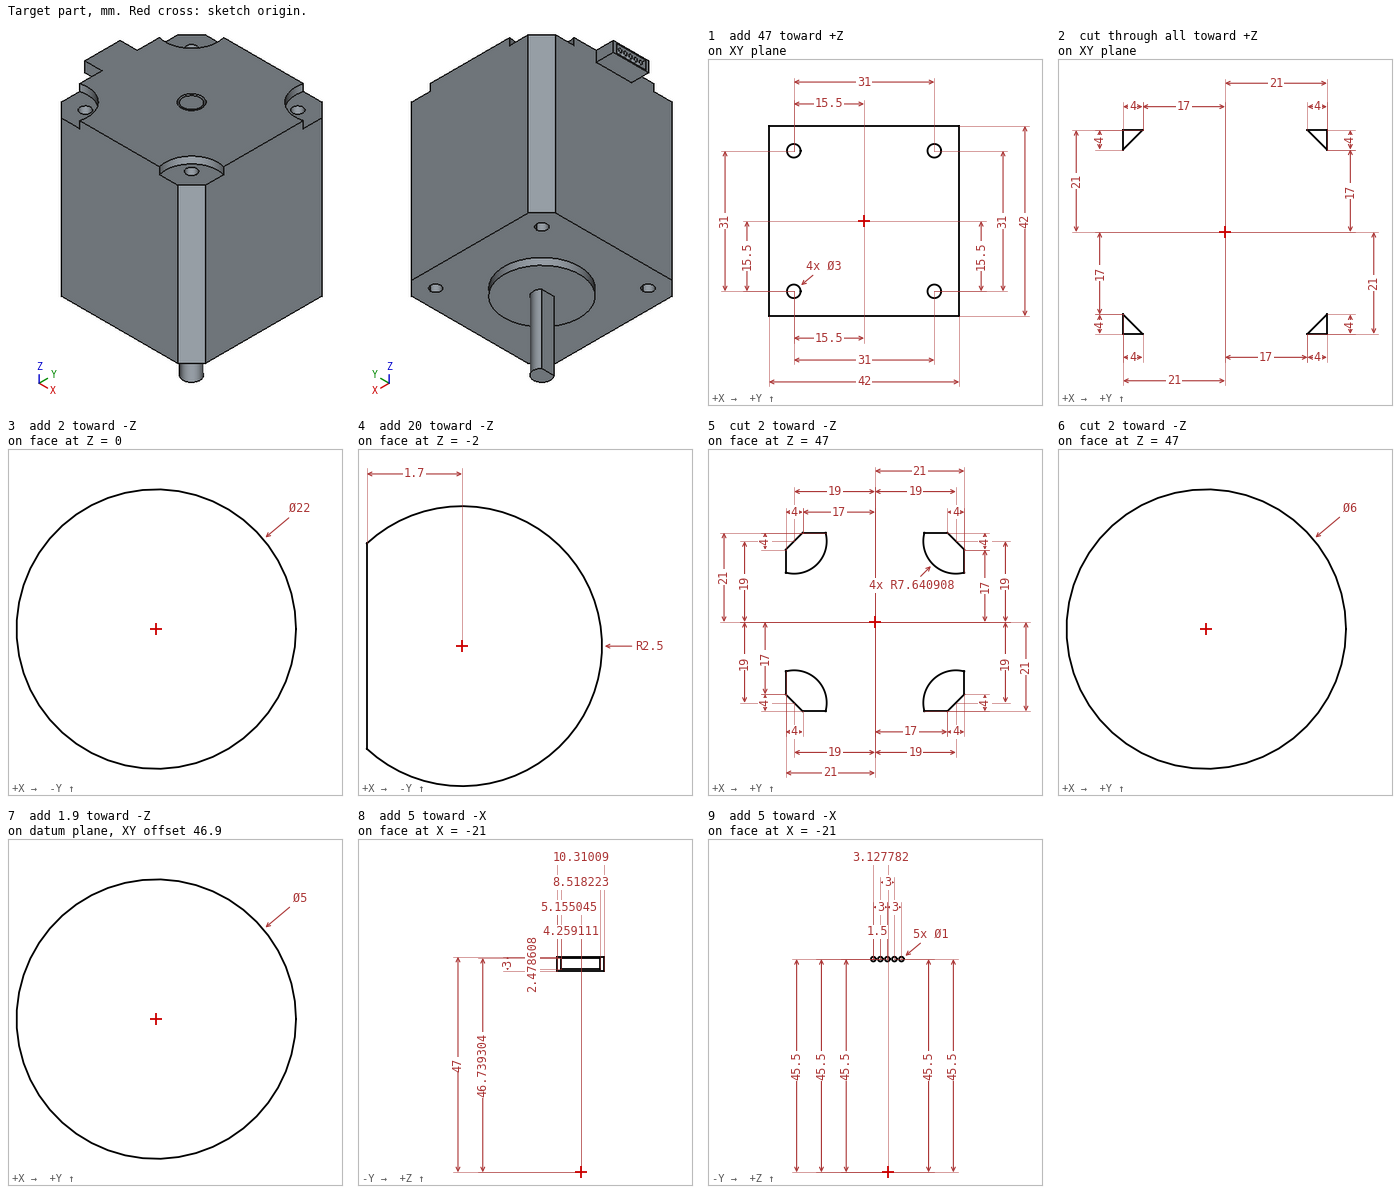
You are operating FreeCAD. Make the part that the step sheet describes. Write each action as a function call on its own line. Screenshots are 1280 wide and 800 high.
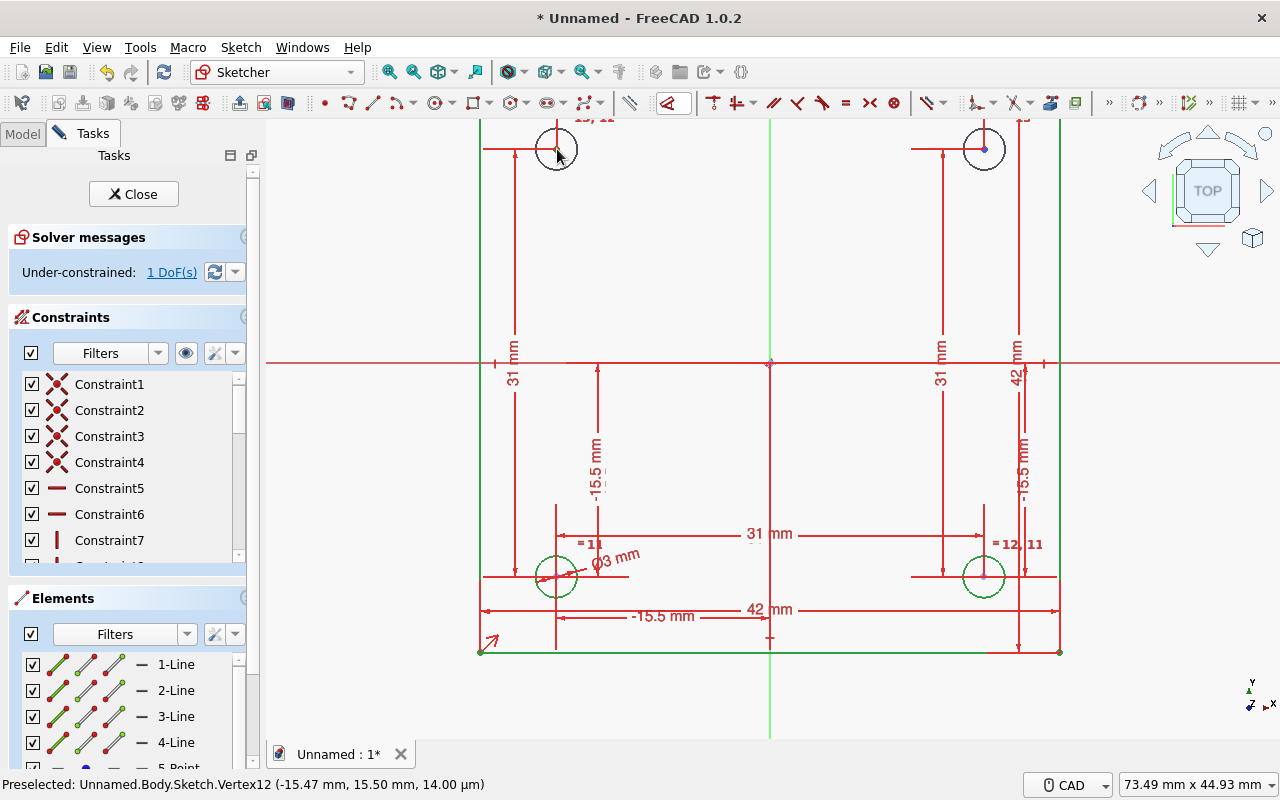
key(l)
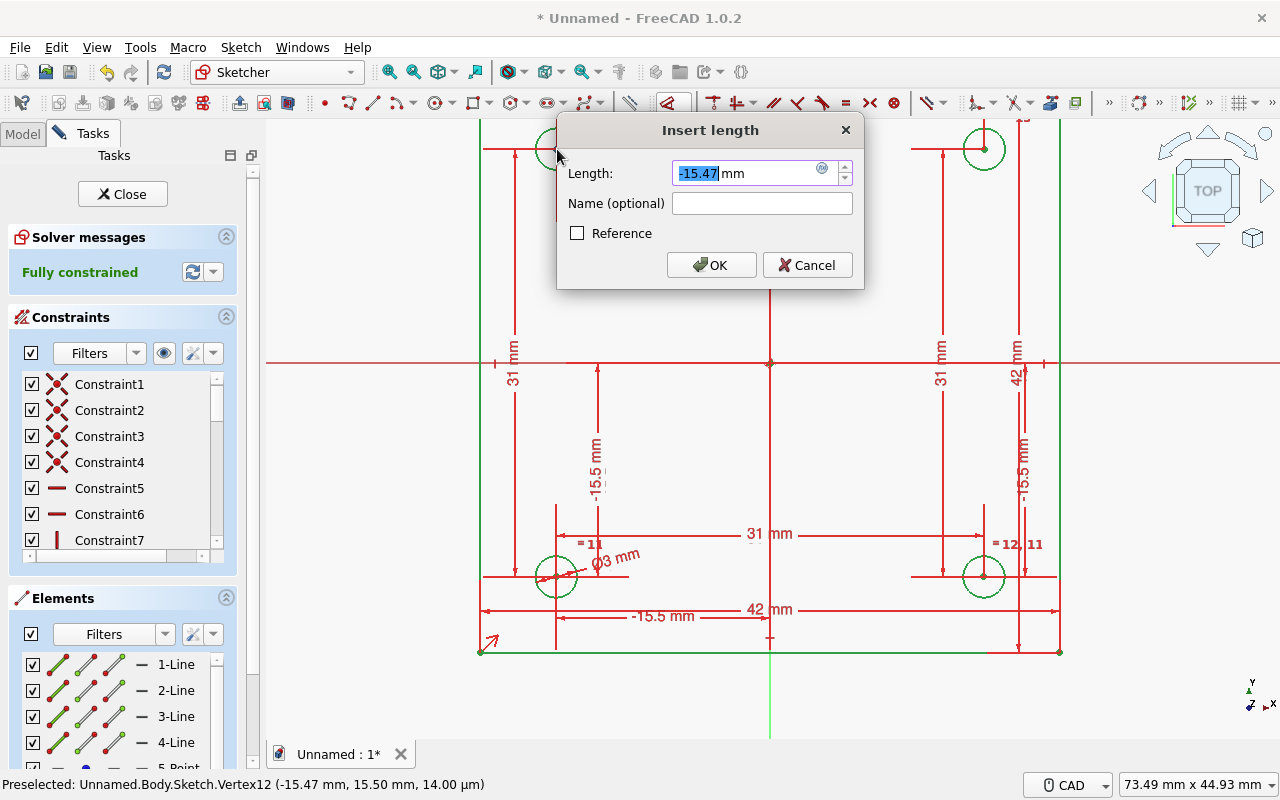
text(-15.5)
key(Return)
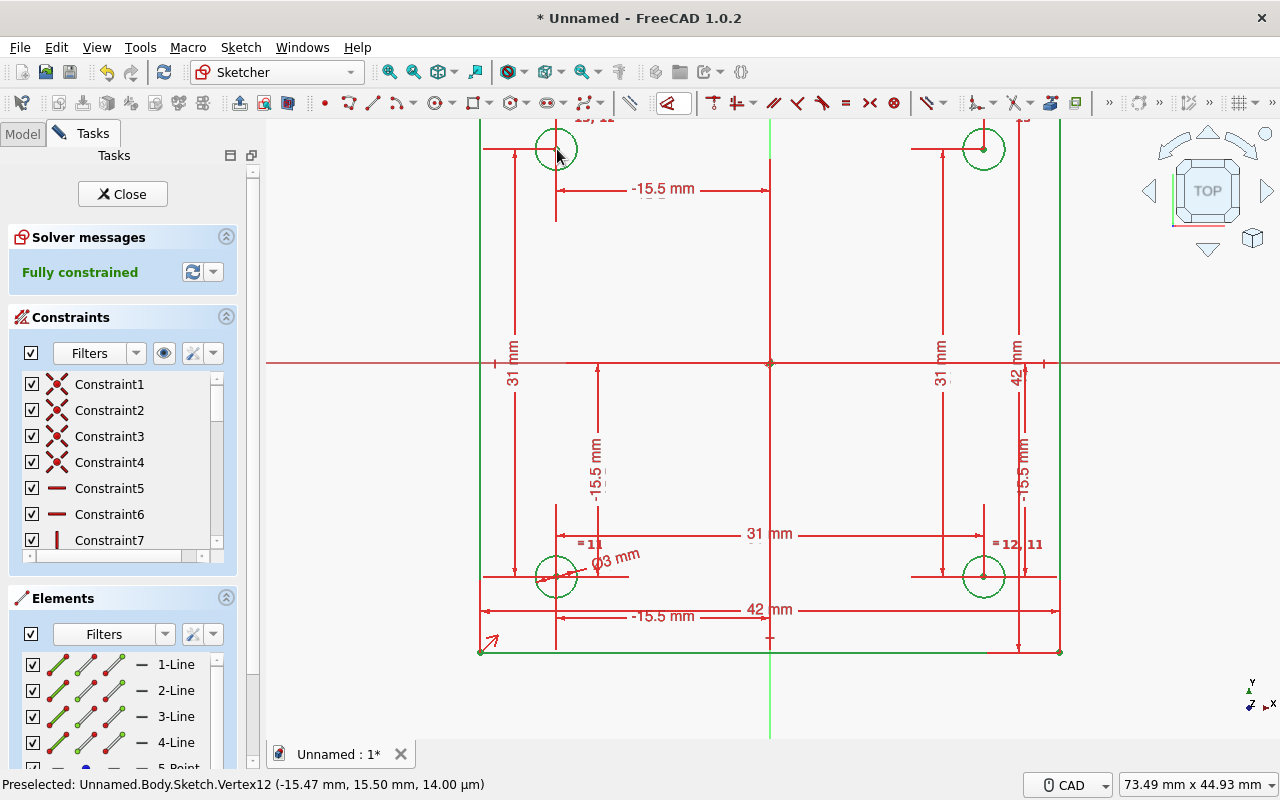
click(123, 194)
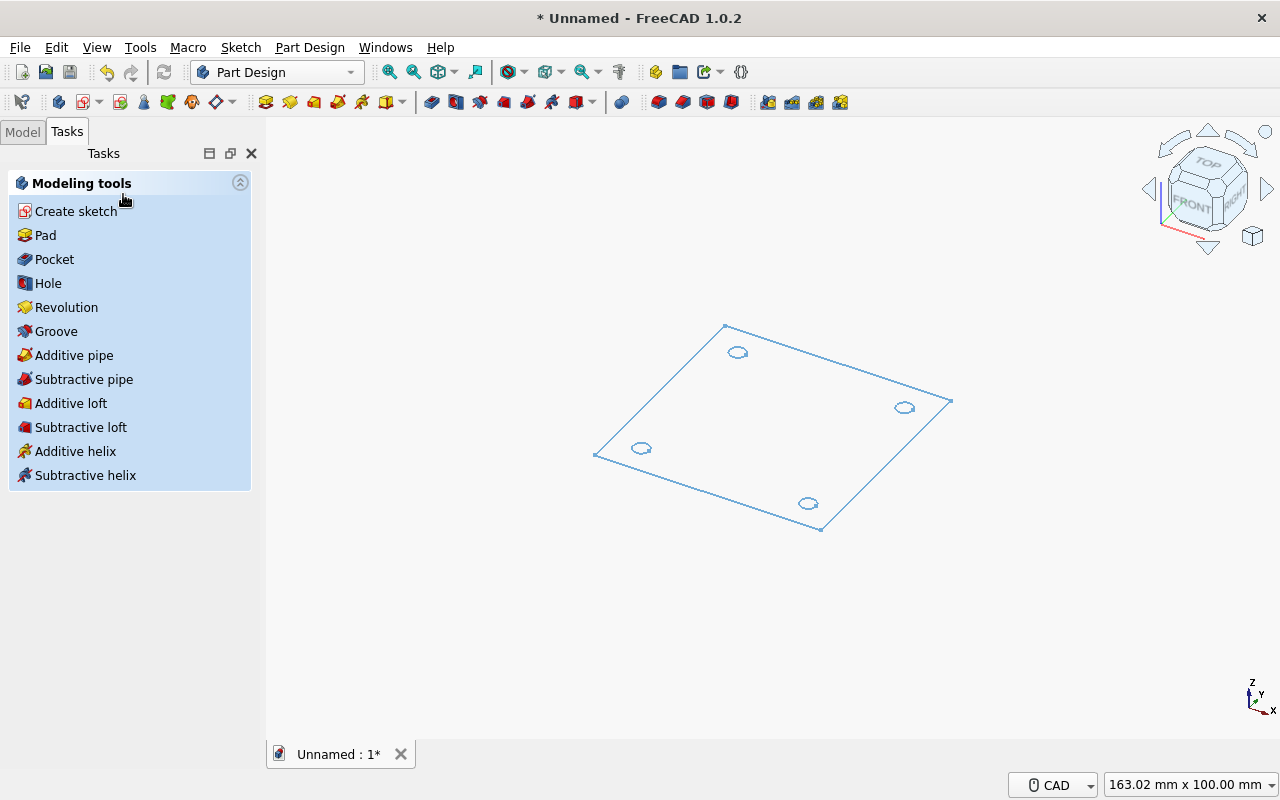
click(266, 102)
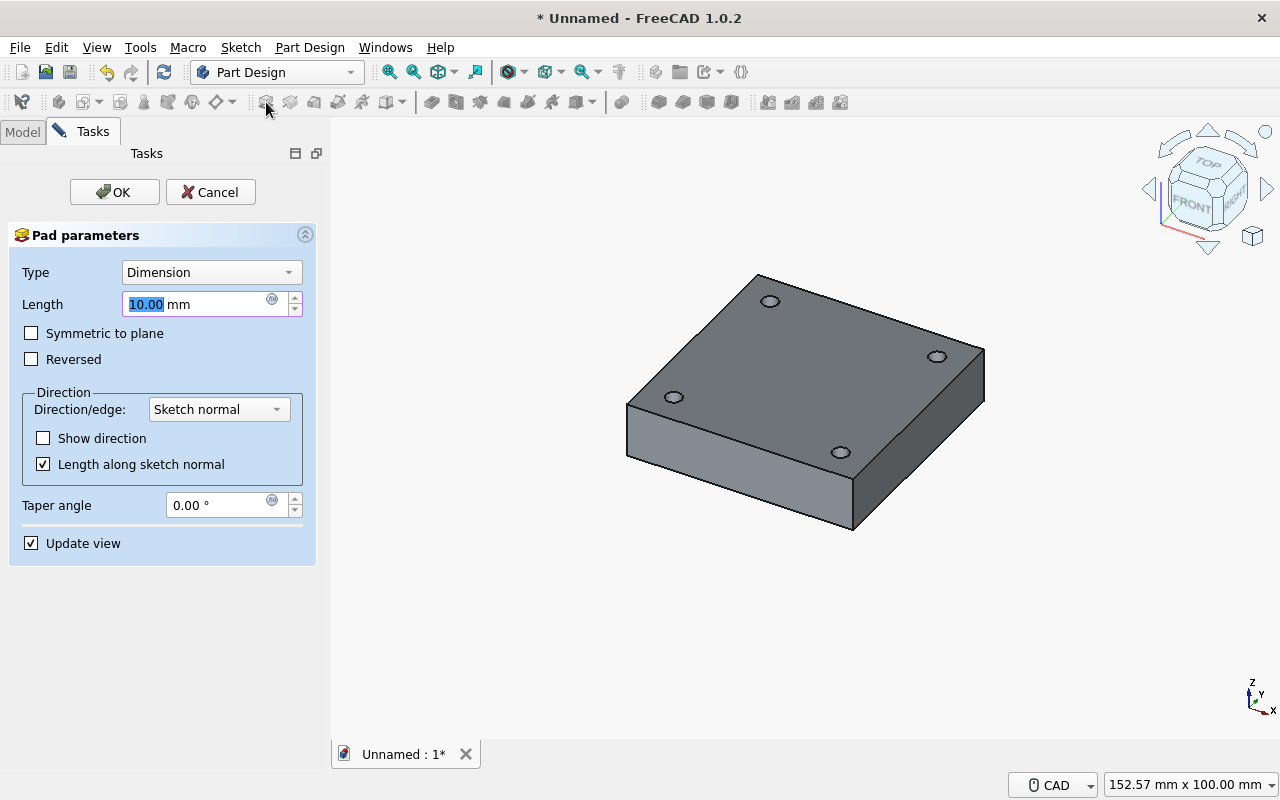
text(47)
key(Tab)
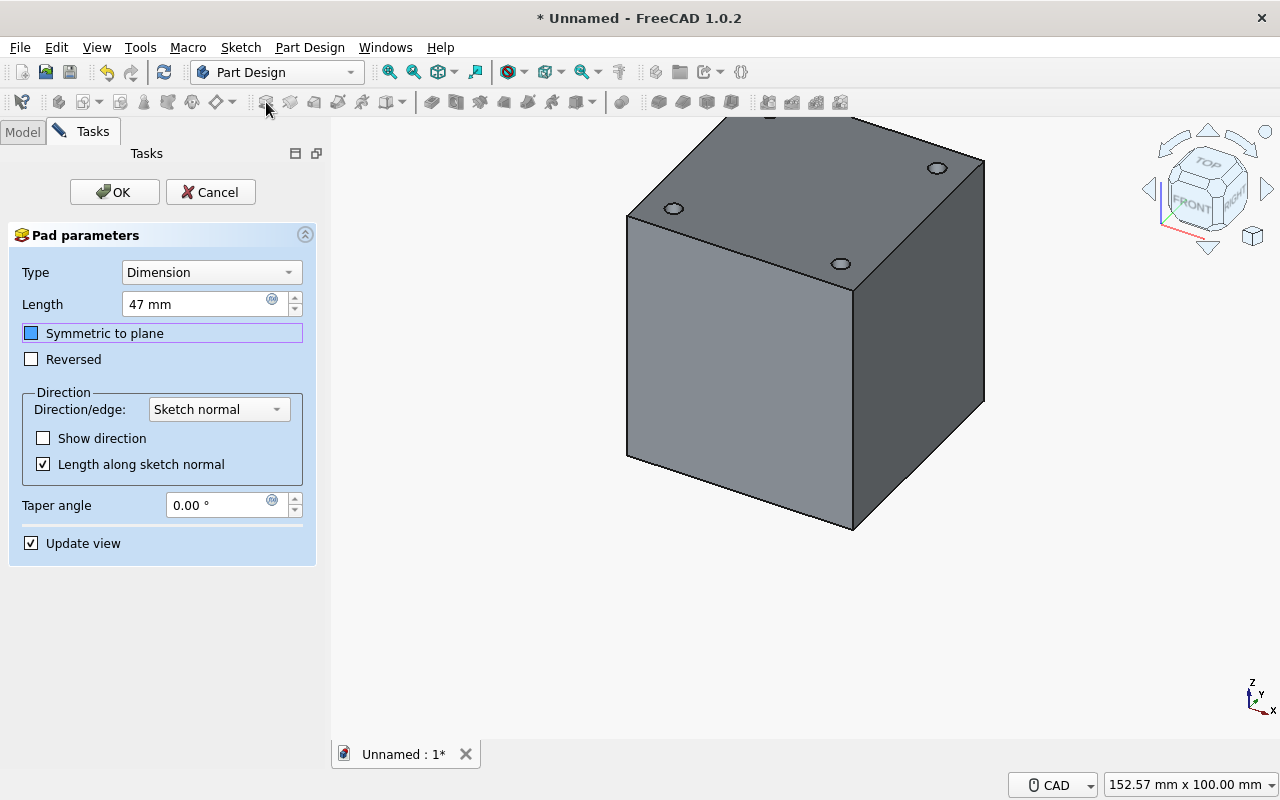
click(115, 192)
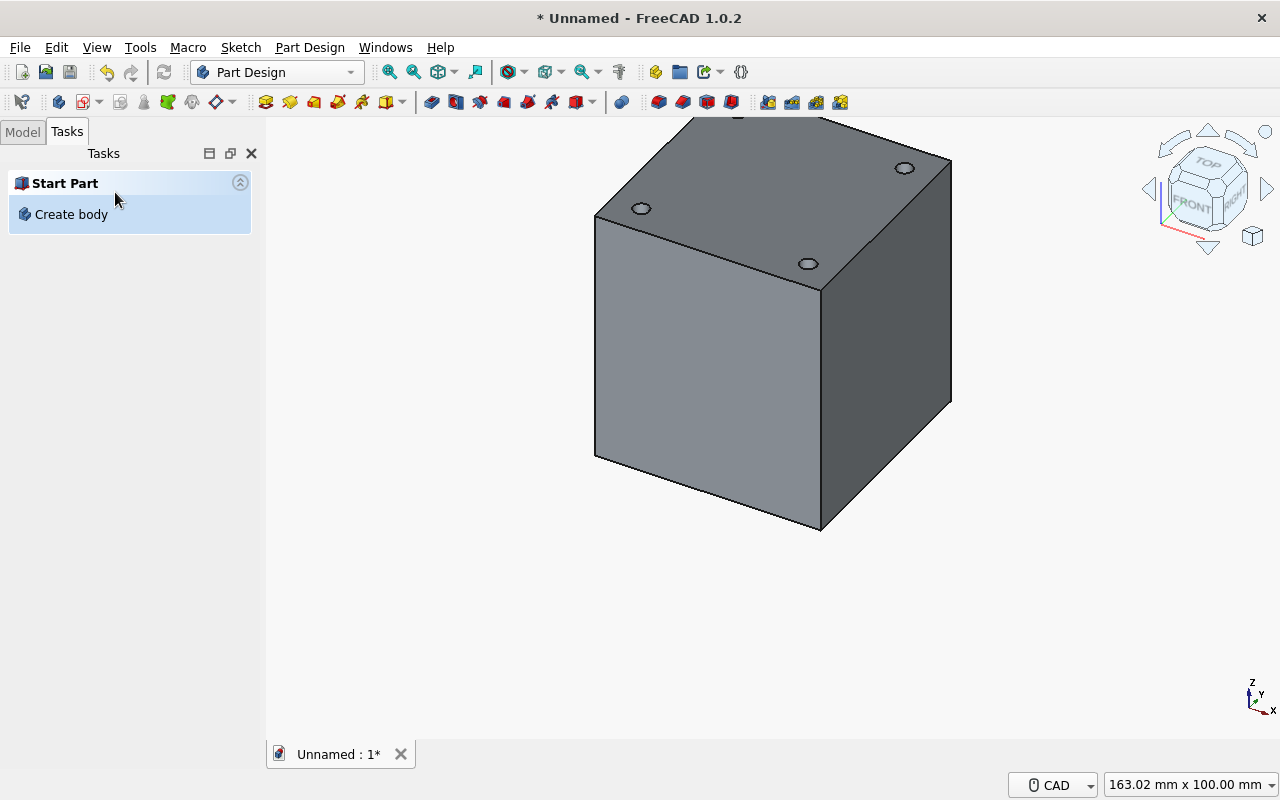
click(390, 72)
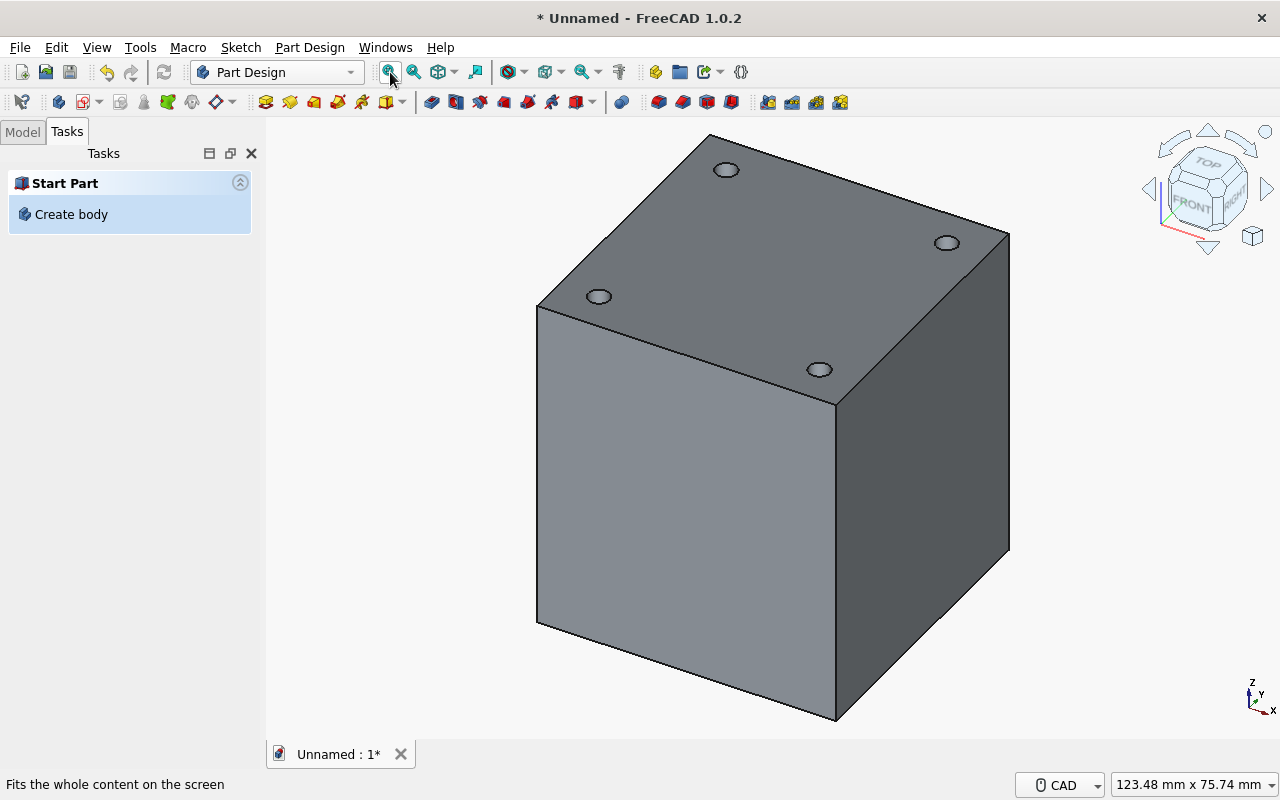
click(84, 102)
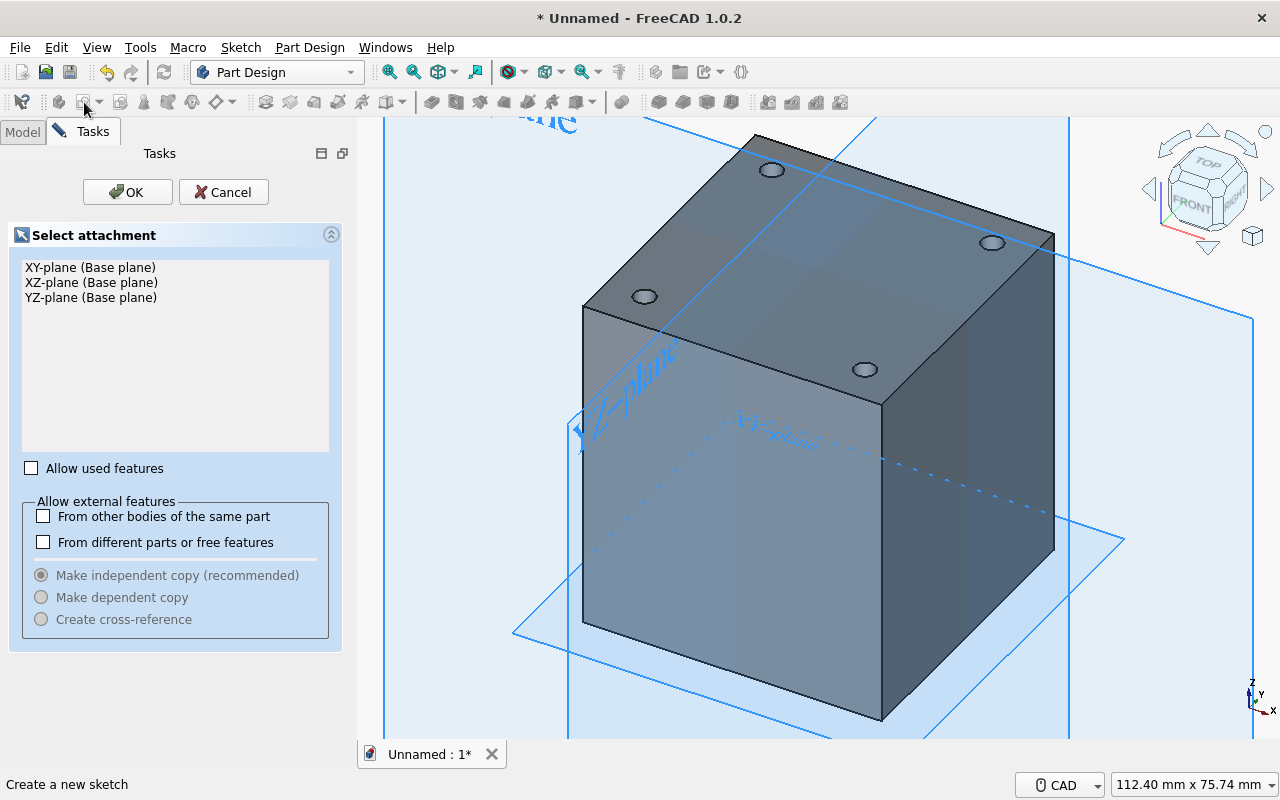
click(82, 268)